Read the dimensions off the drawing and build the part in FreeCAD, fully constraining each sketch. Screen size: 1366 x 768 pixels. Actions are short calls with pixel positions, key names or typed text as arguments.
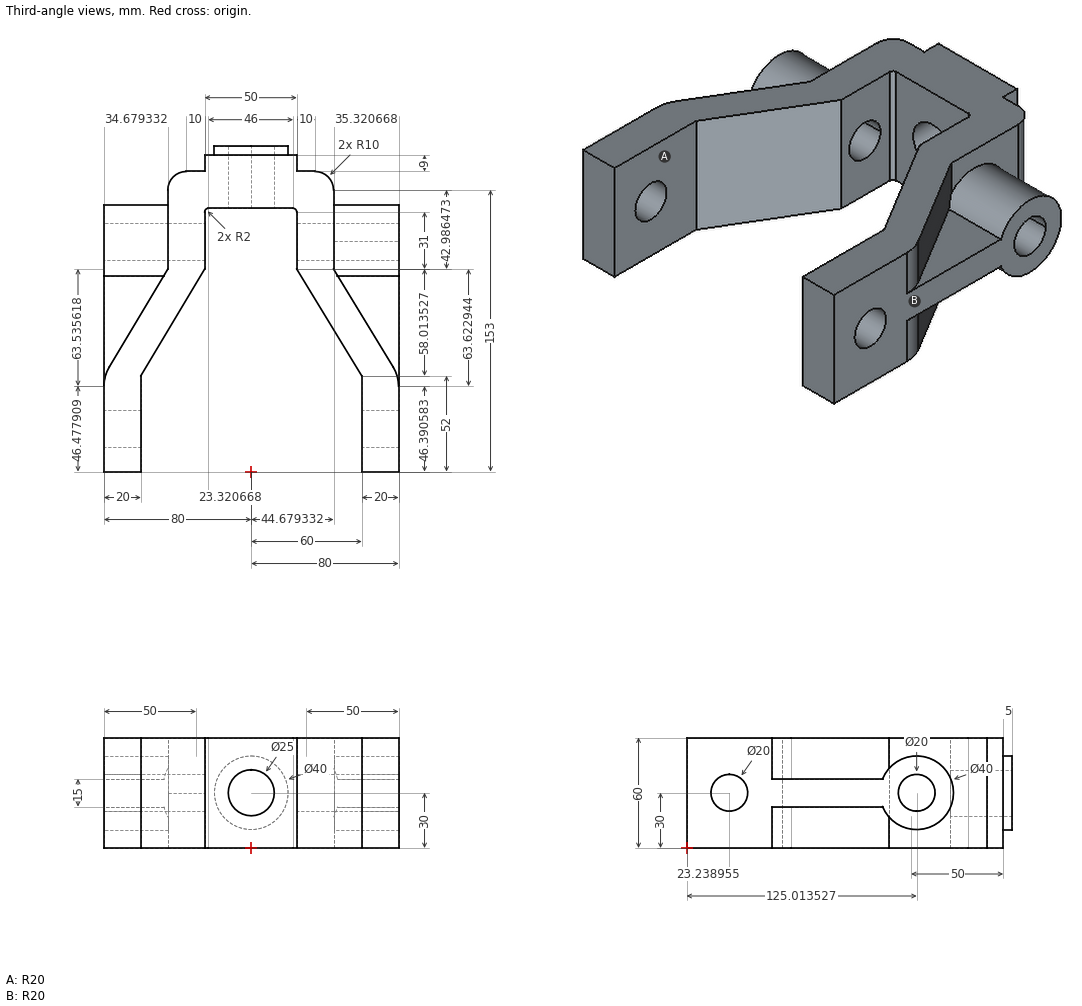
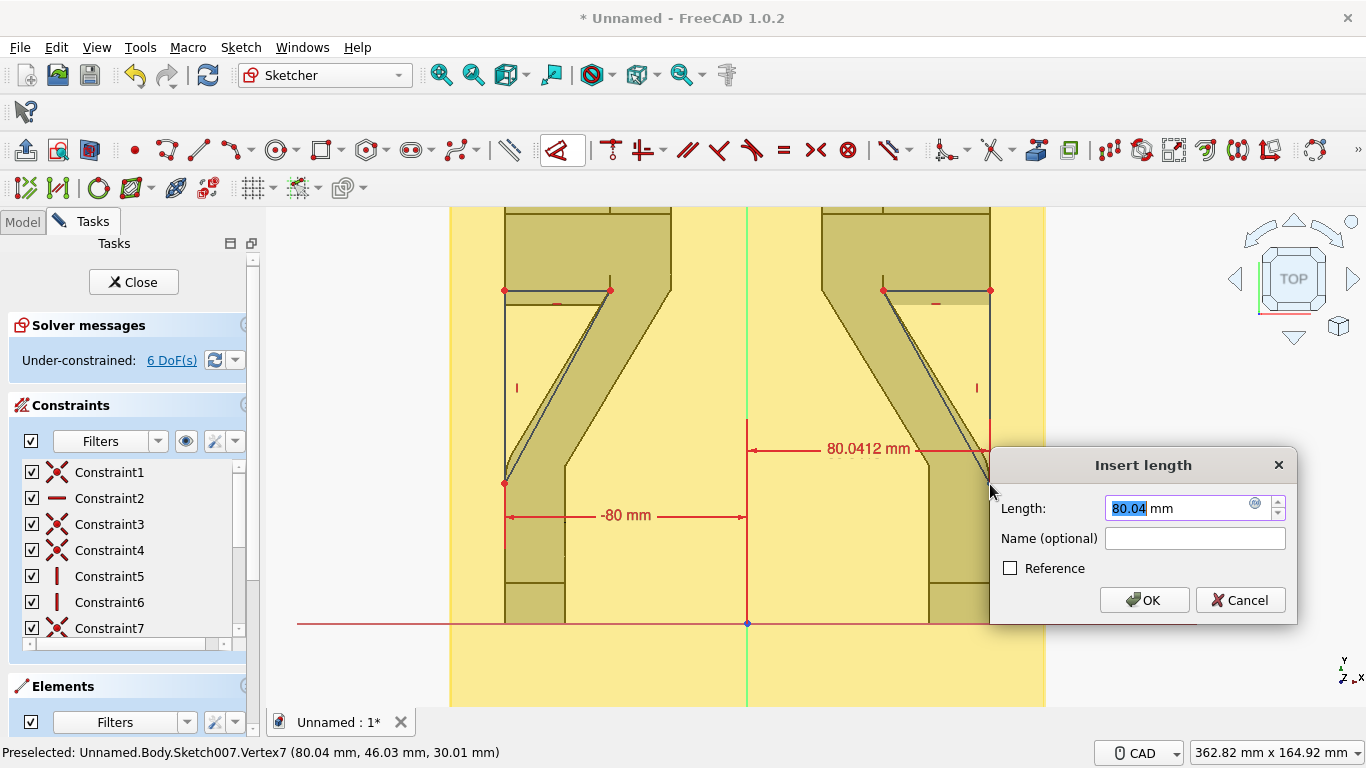
text(80)
key(Return)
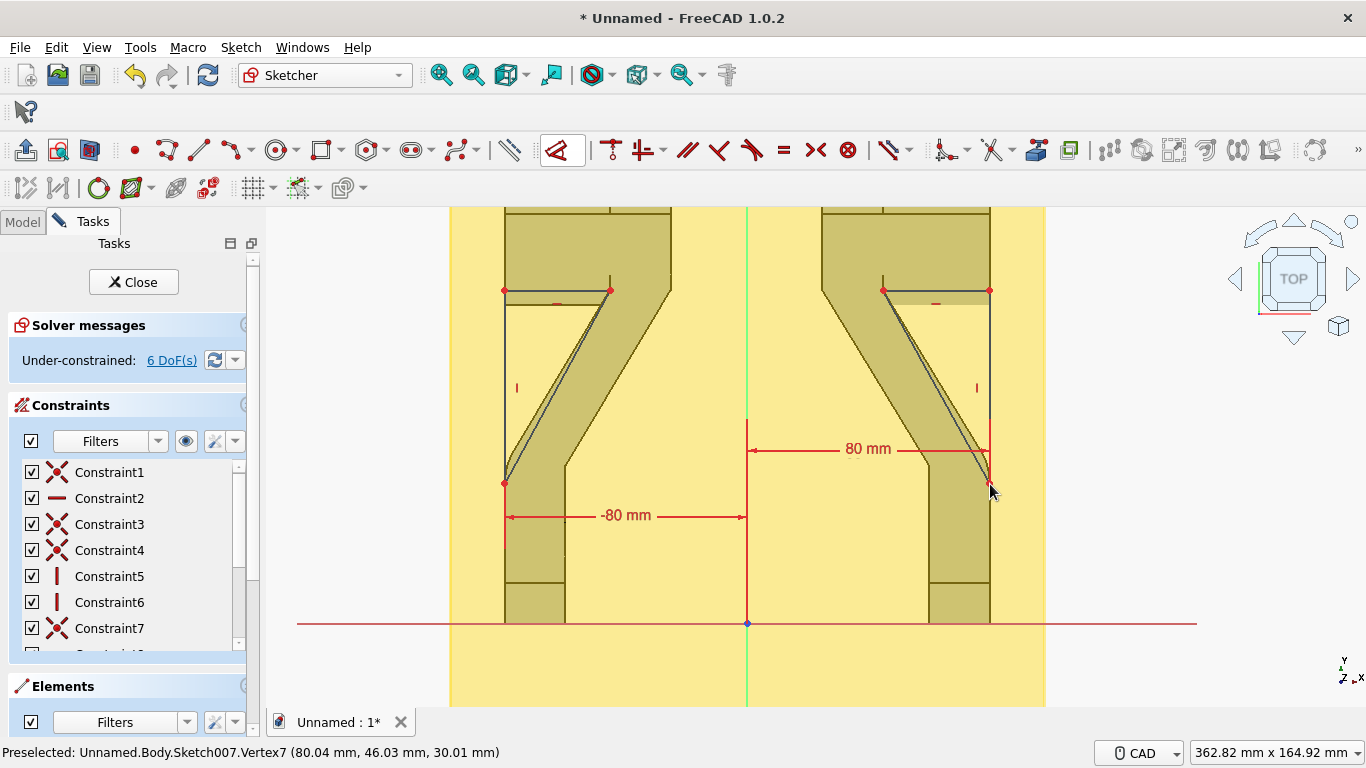
click(578, 291)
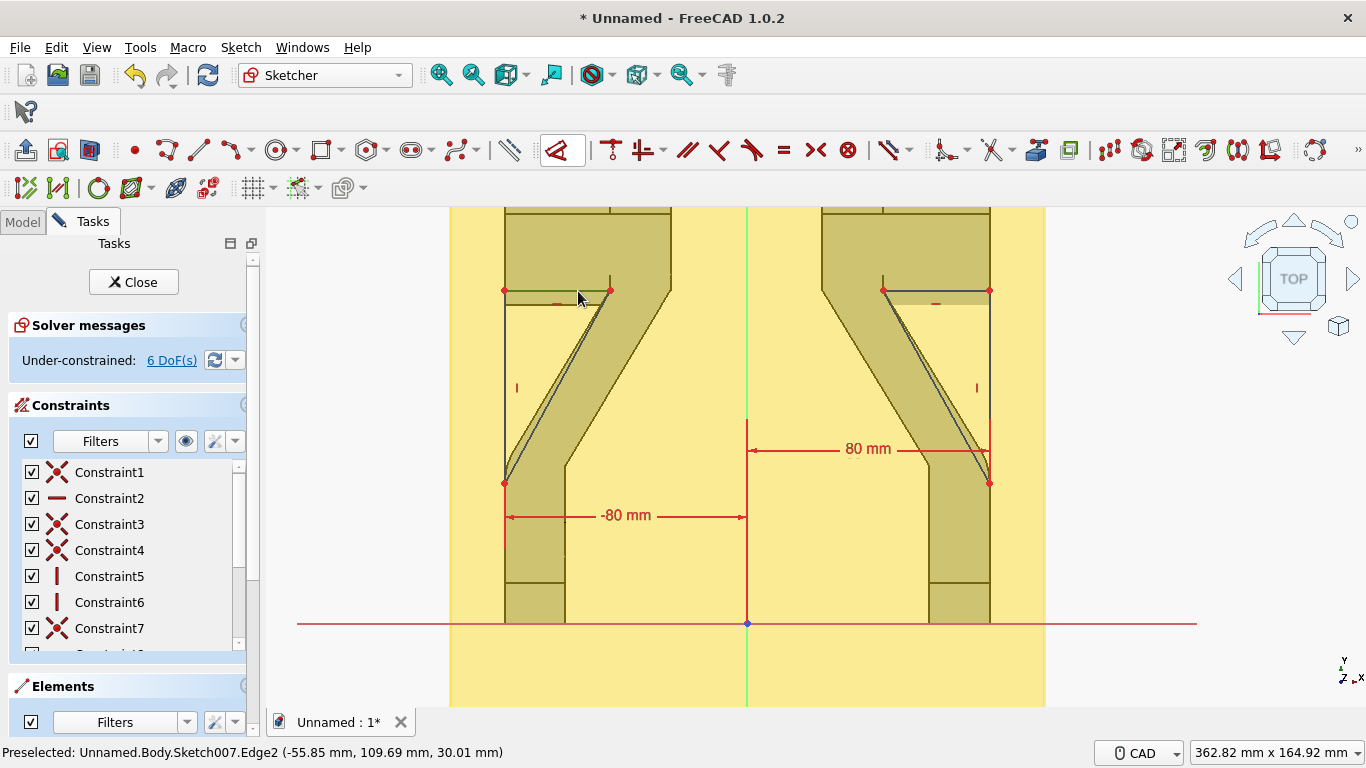
key(l)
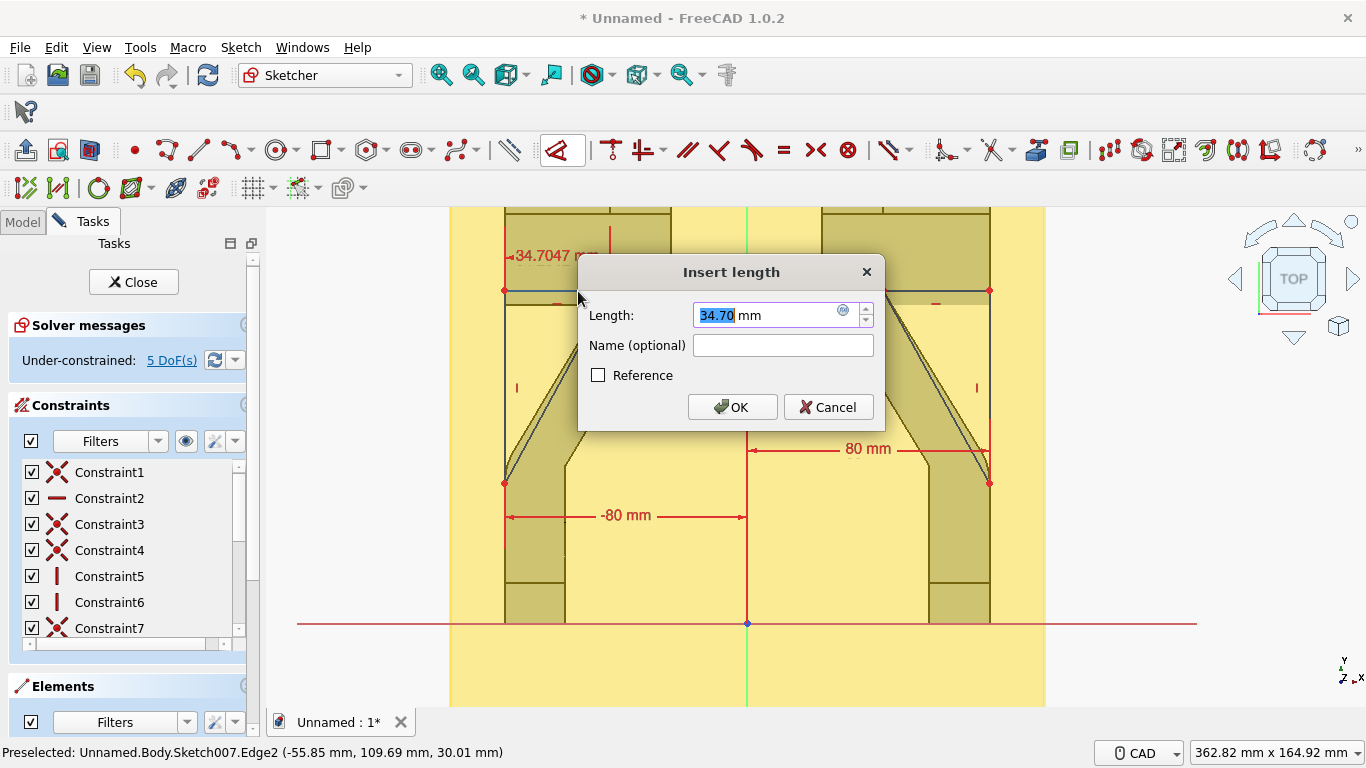
text(34.679332)
key(Return)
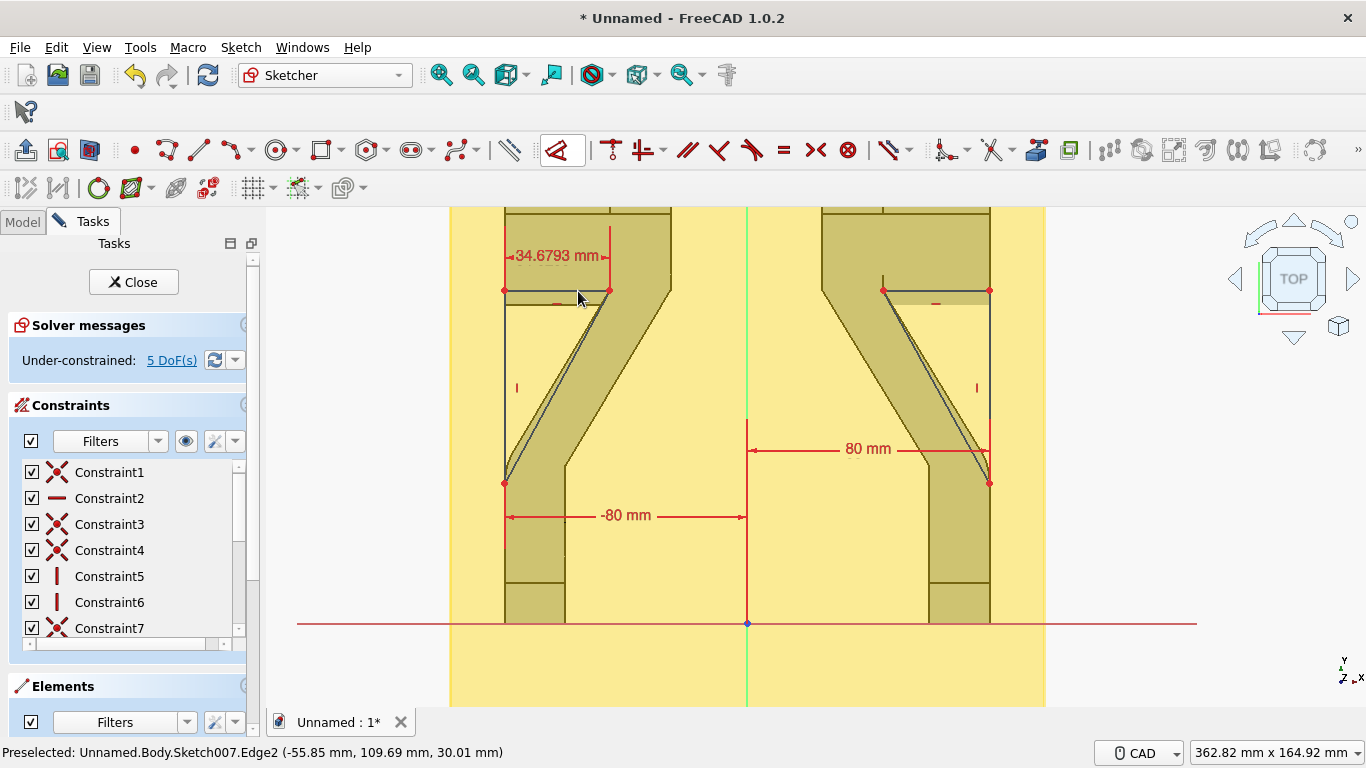
click(505, 349)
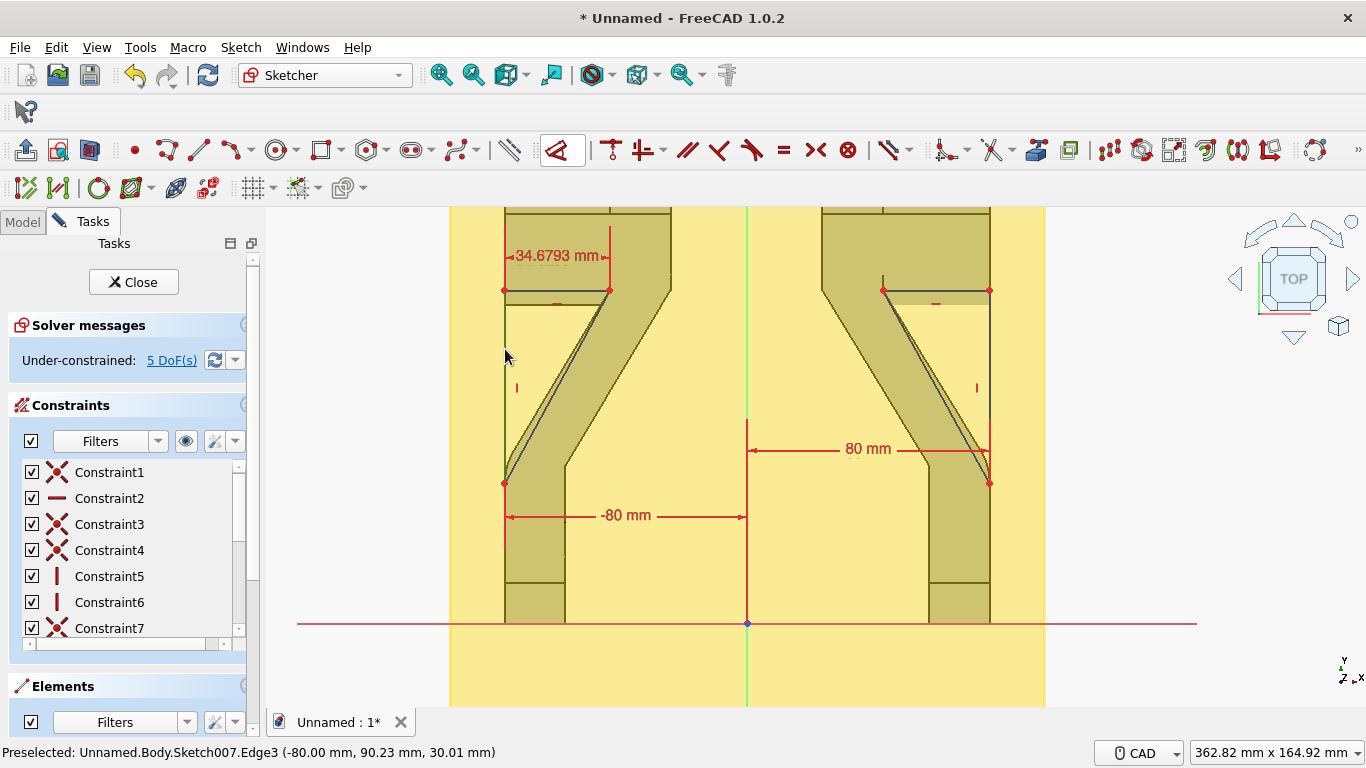
key(i)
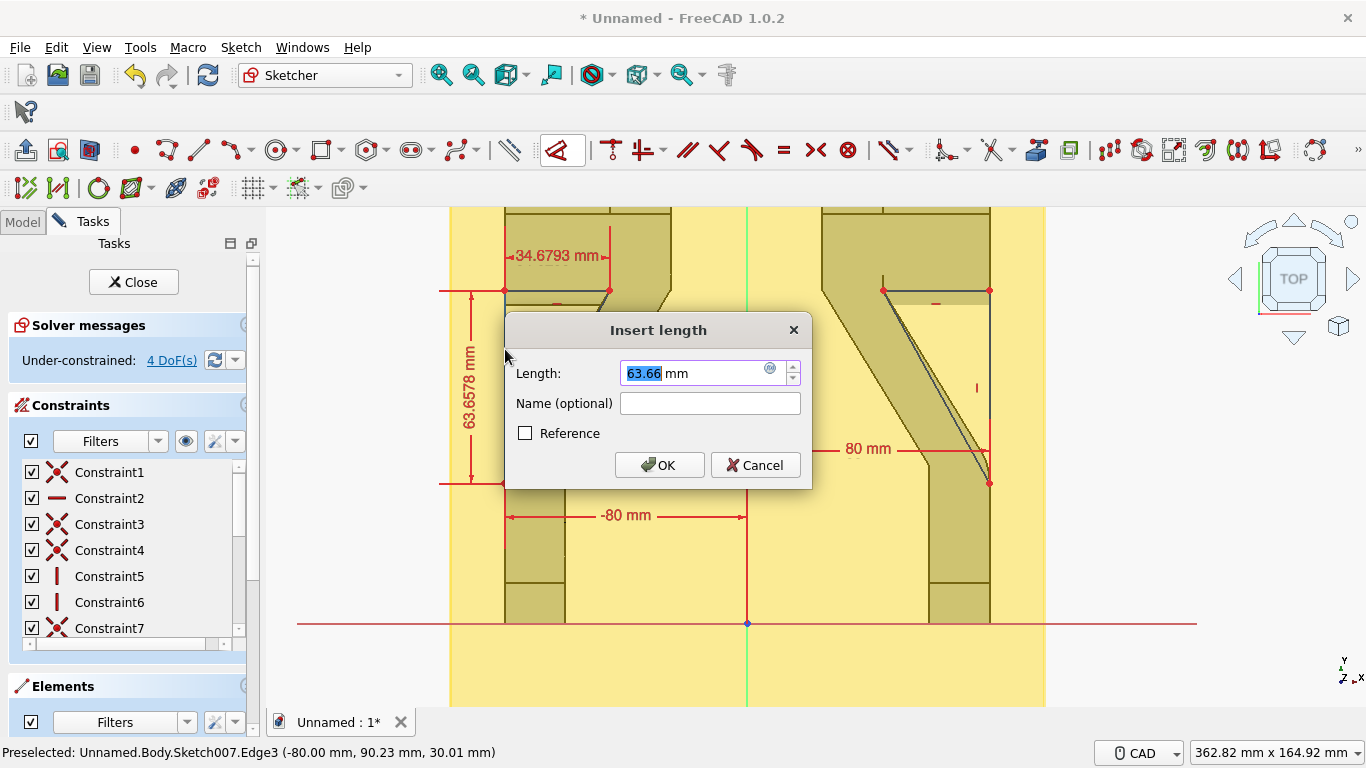
text(63.535618)
key(Return)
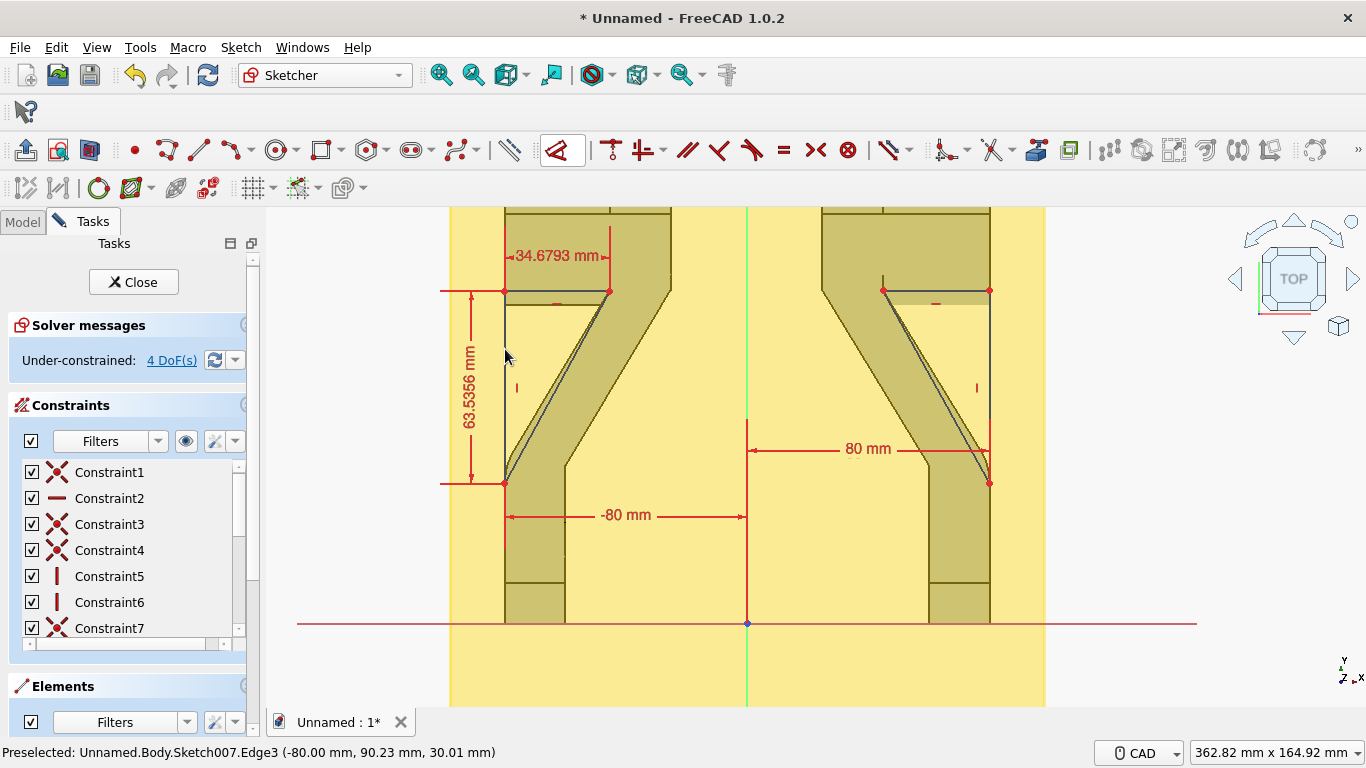
click(990, 426)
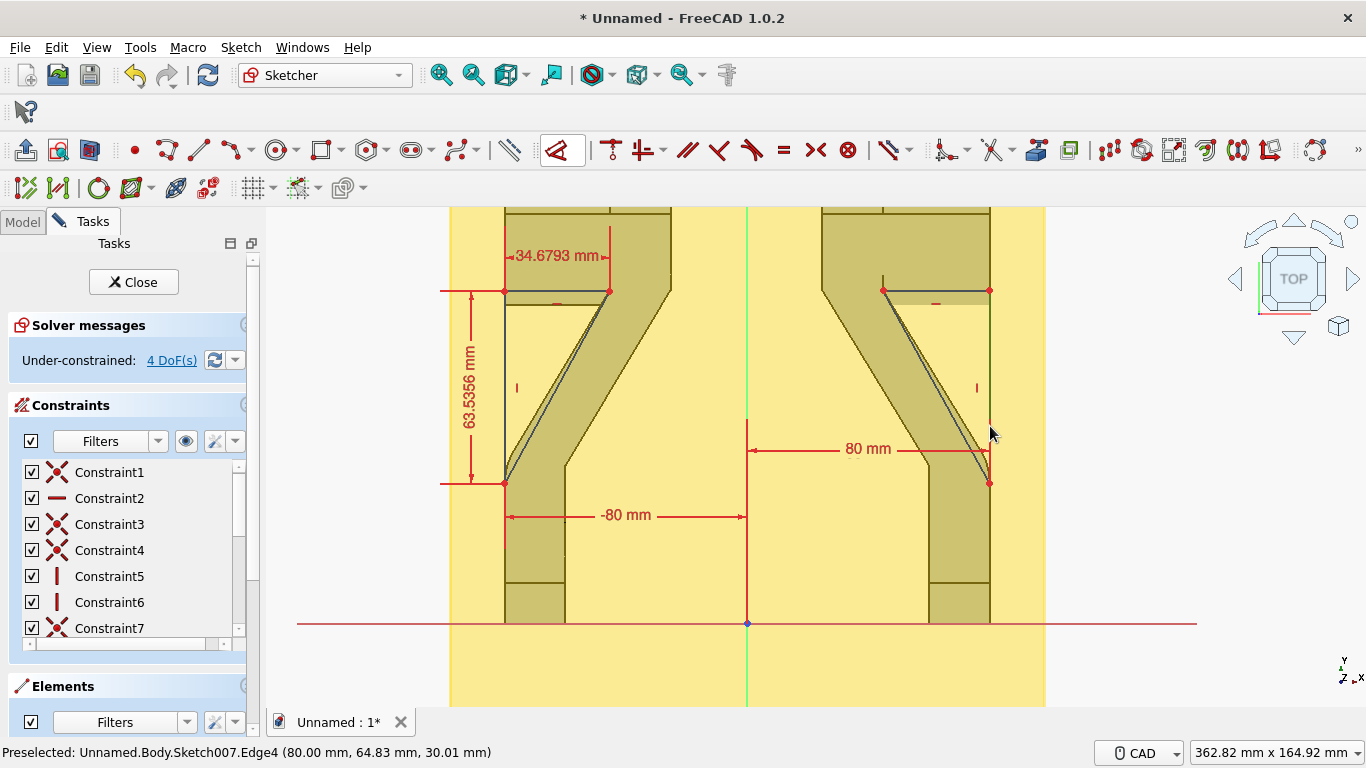
key(i)